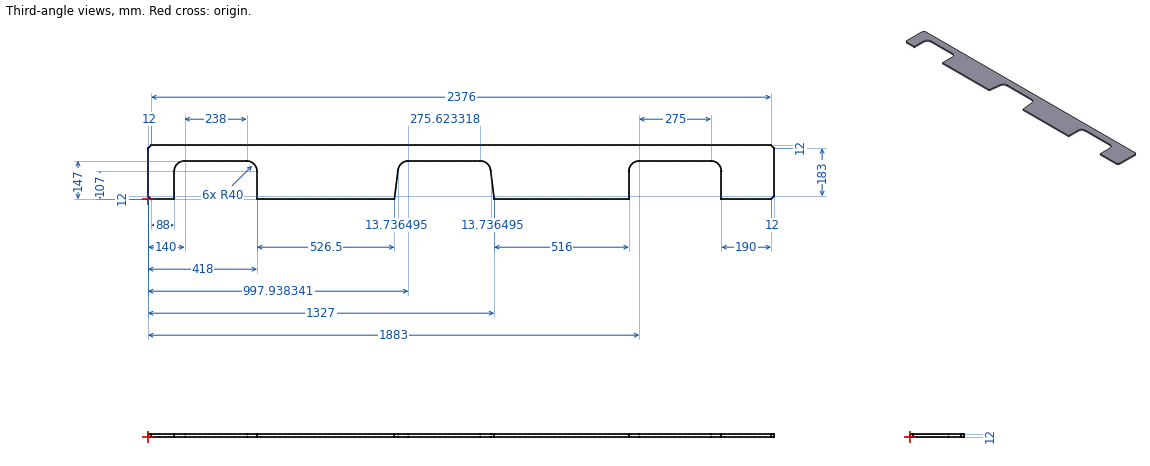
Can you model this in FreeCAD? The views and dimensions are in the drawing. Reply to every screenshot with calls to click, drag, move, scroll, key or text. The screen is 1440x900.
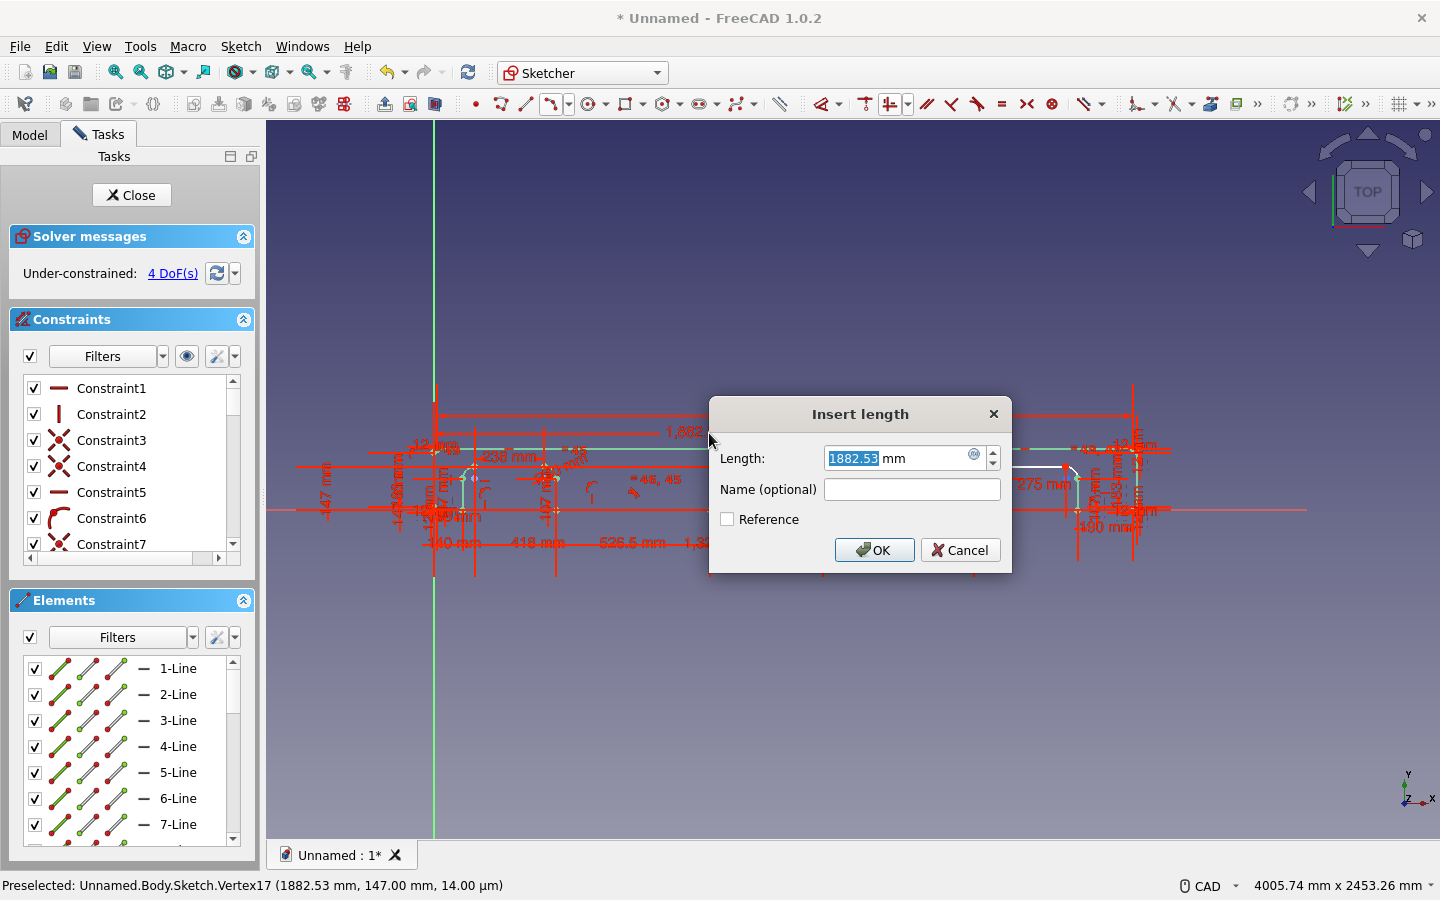
text(1883)
key(Return)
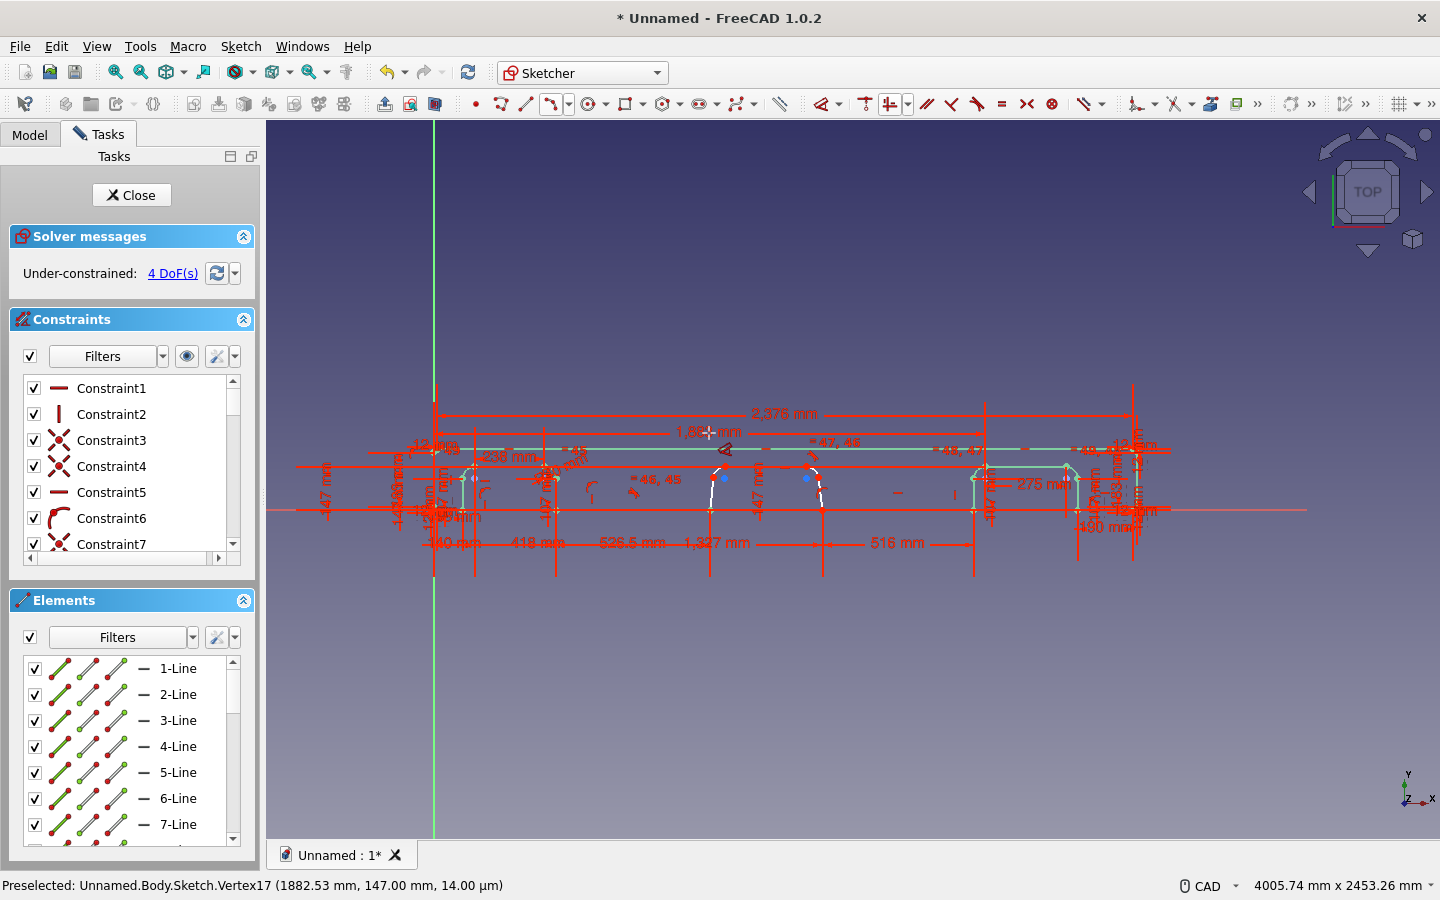
click(750, 467)
click(795, 525)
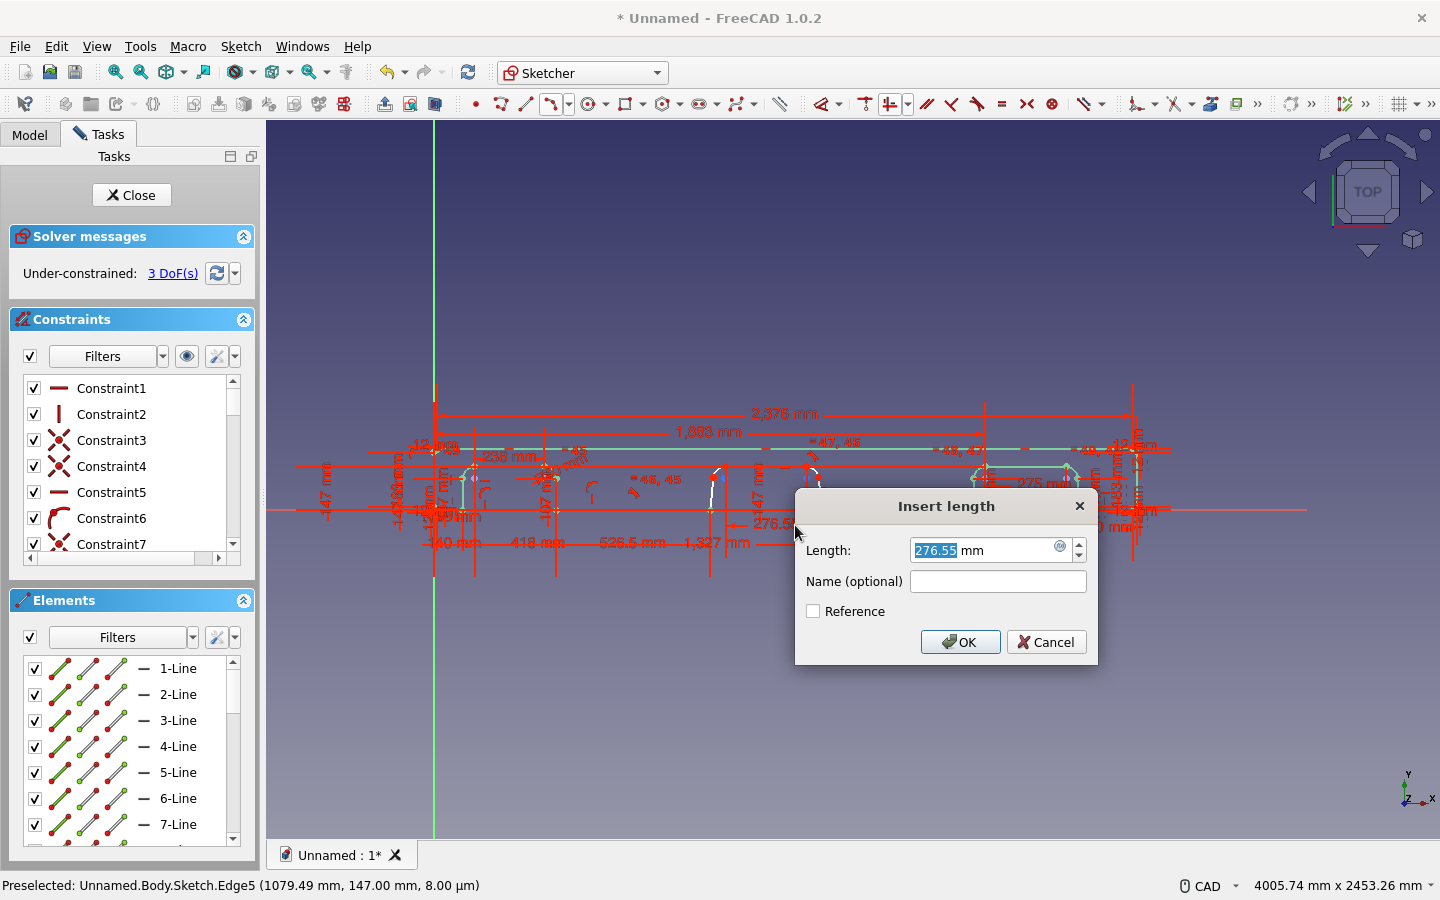
text(275.623318)
key(Return)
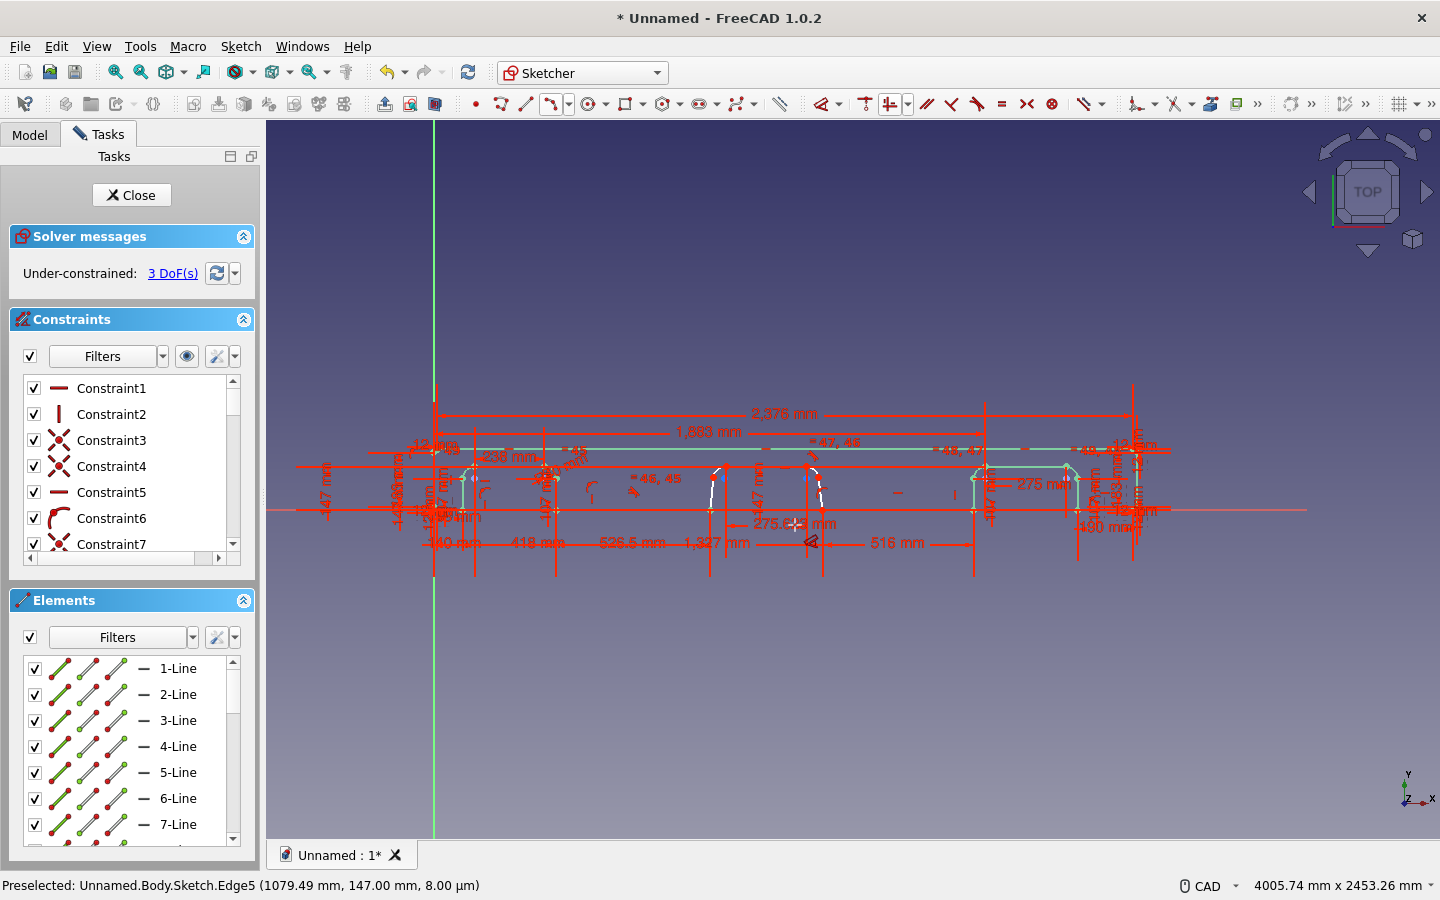
scroll(711, 500, up, 12)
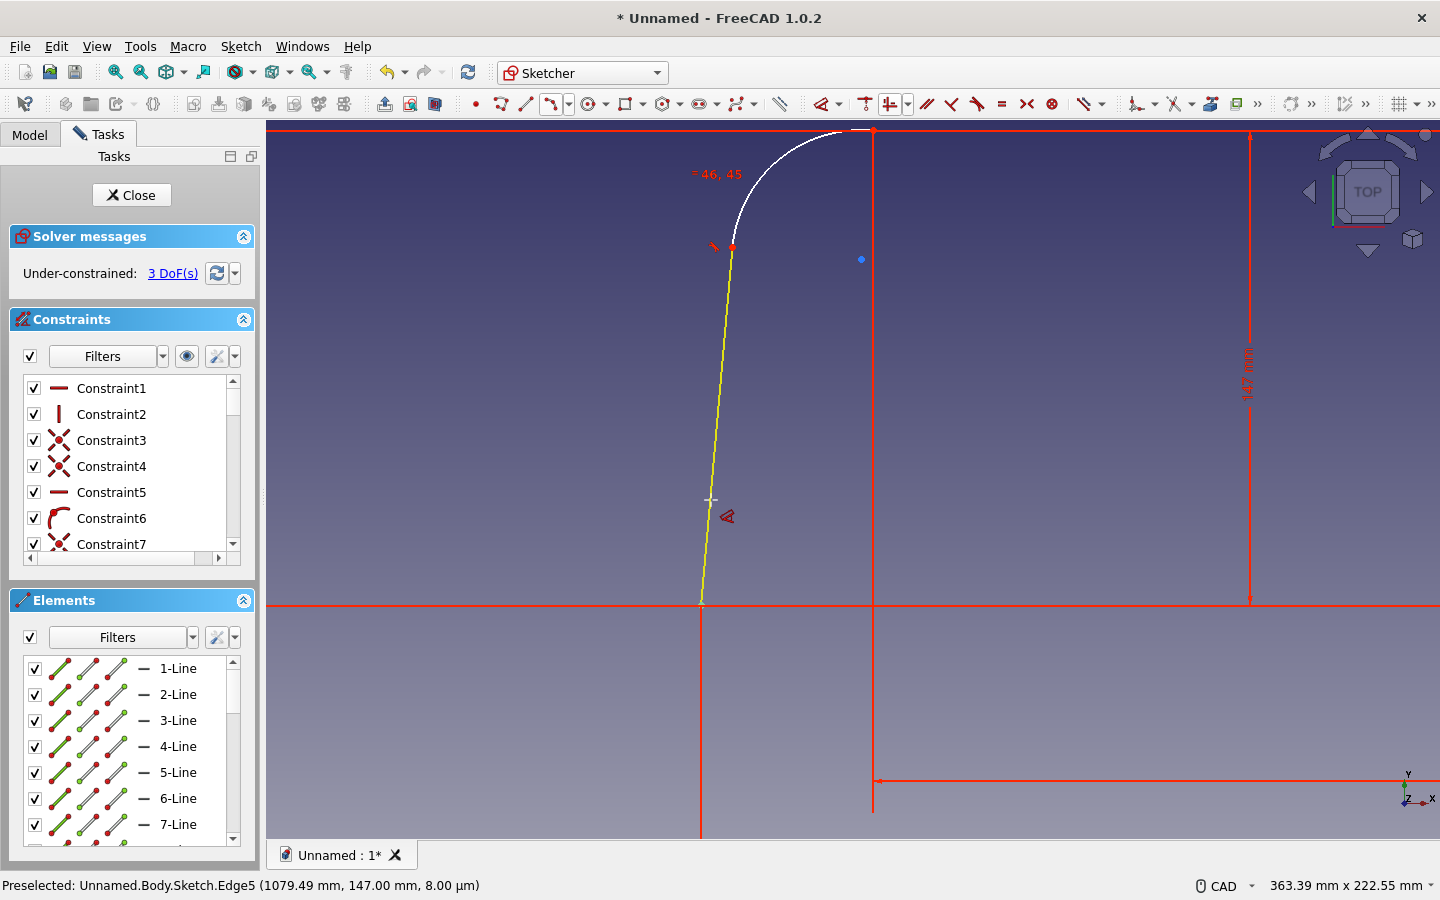
click(710, 498)
click(717, 640)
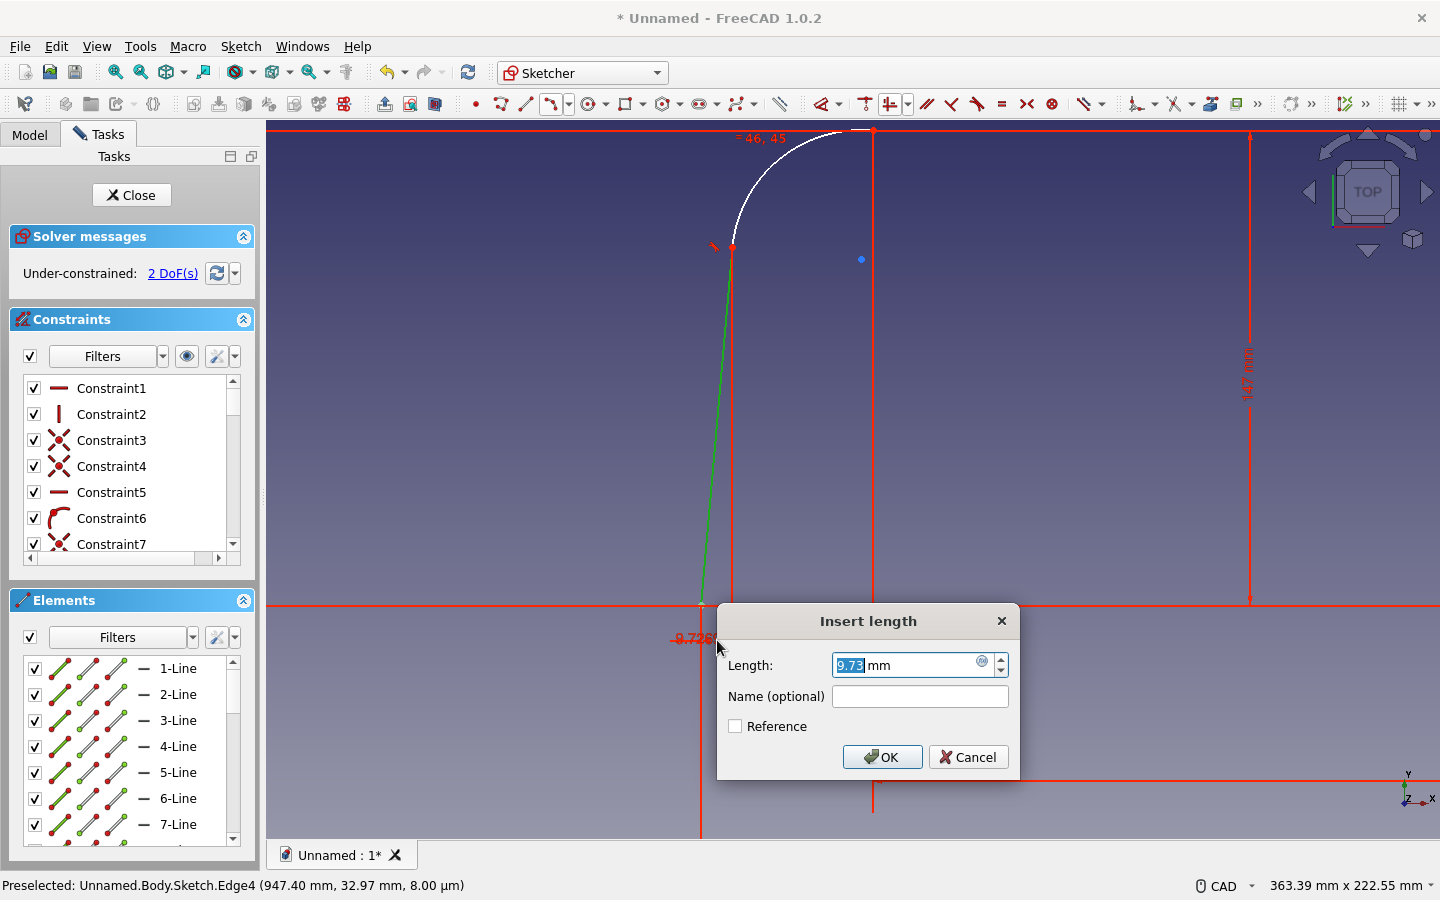
text(13.736495)
key(Return)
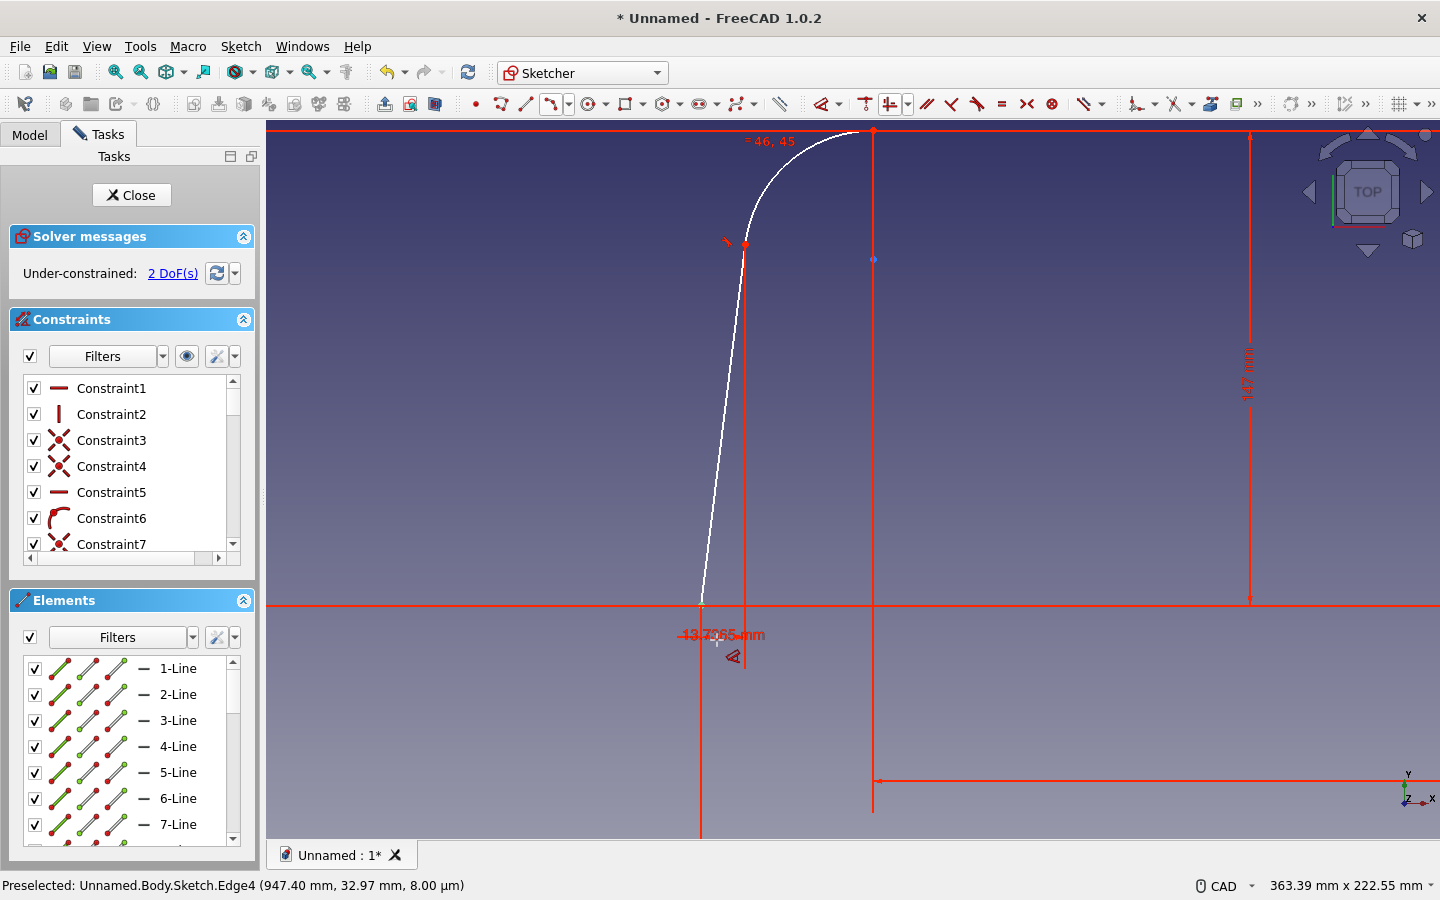
scroll(710, 500, down, 12)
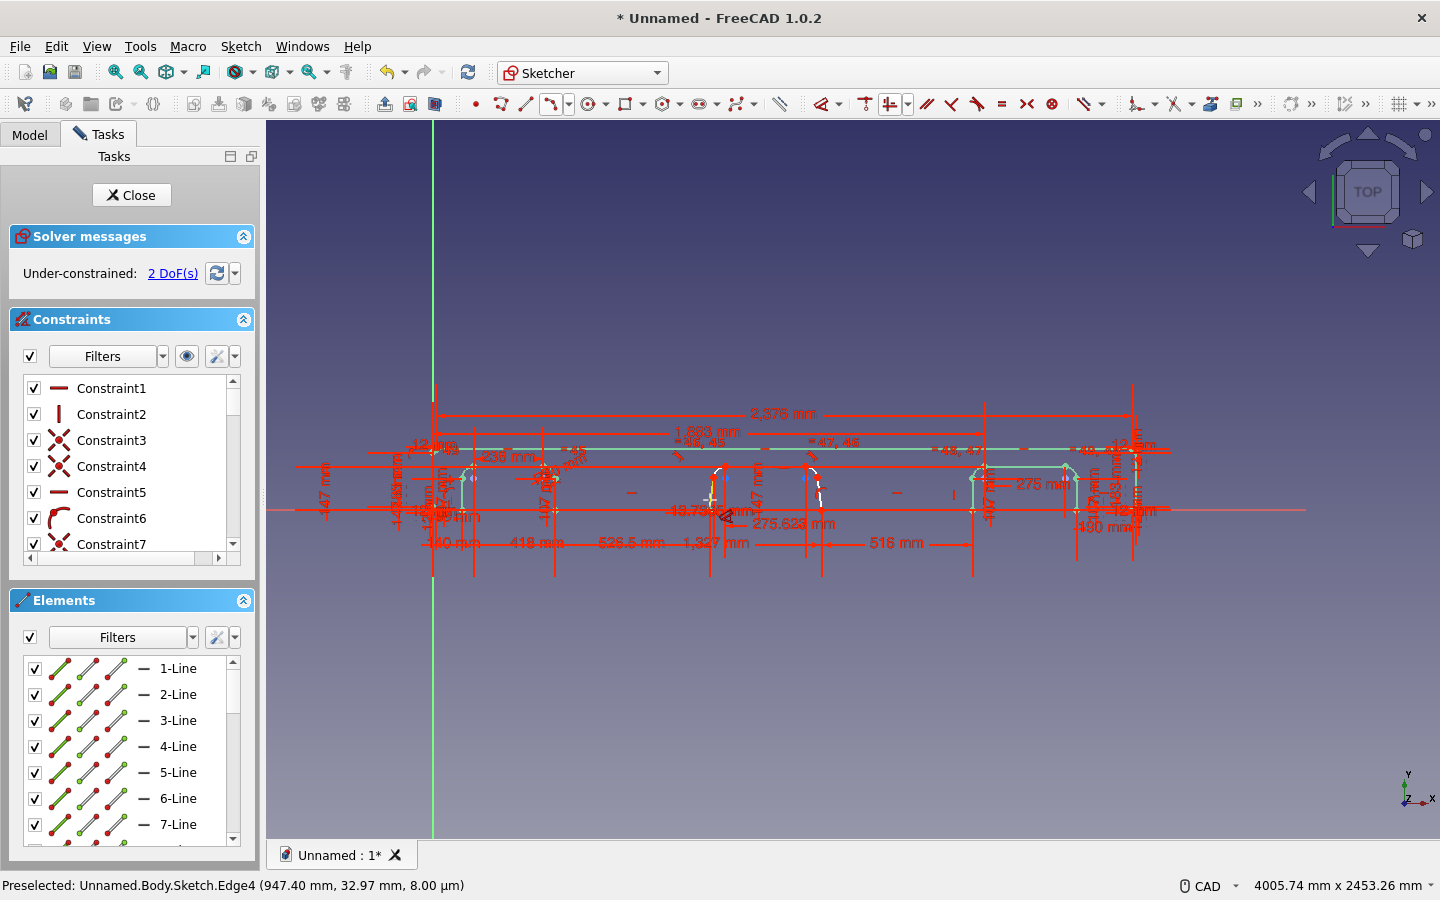
scroll(819, 487, up, 12)